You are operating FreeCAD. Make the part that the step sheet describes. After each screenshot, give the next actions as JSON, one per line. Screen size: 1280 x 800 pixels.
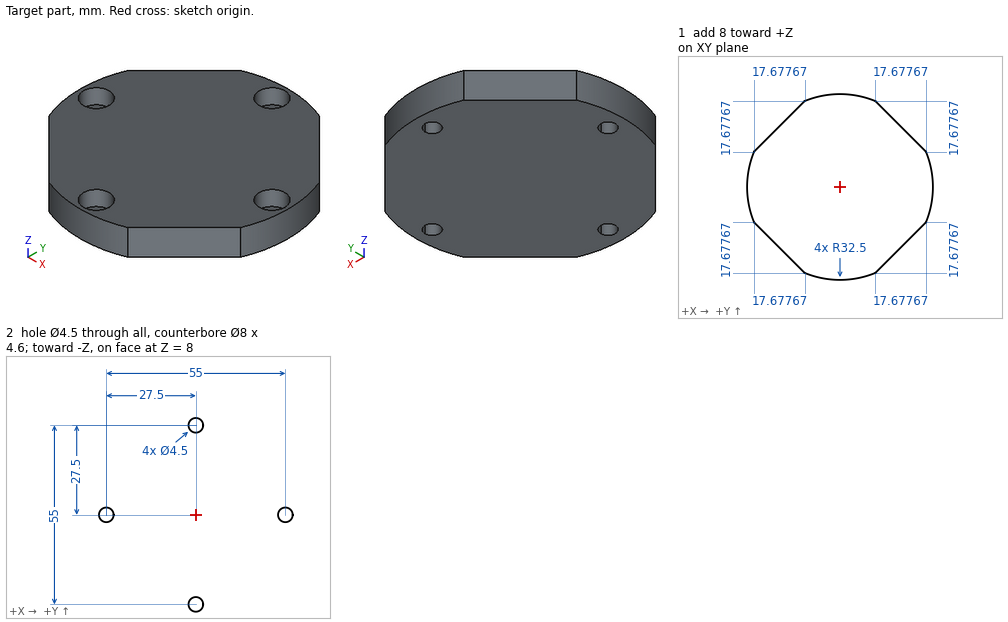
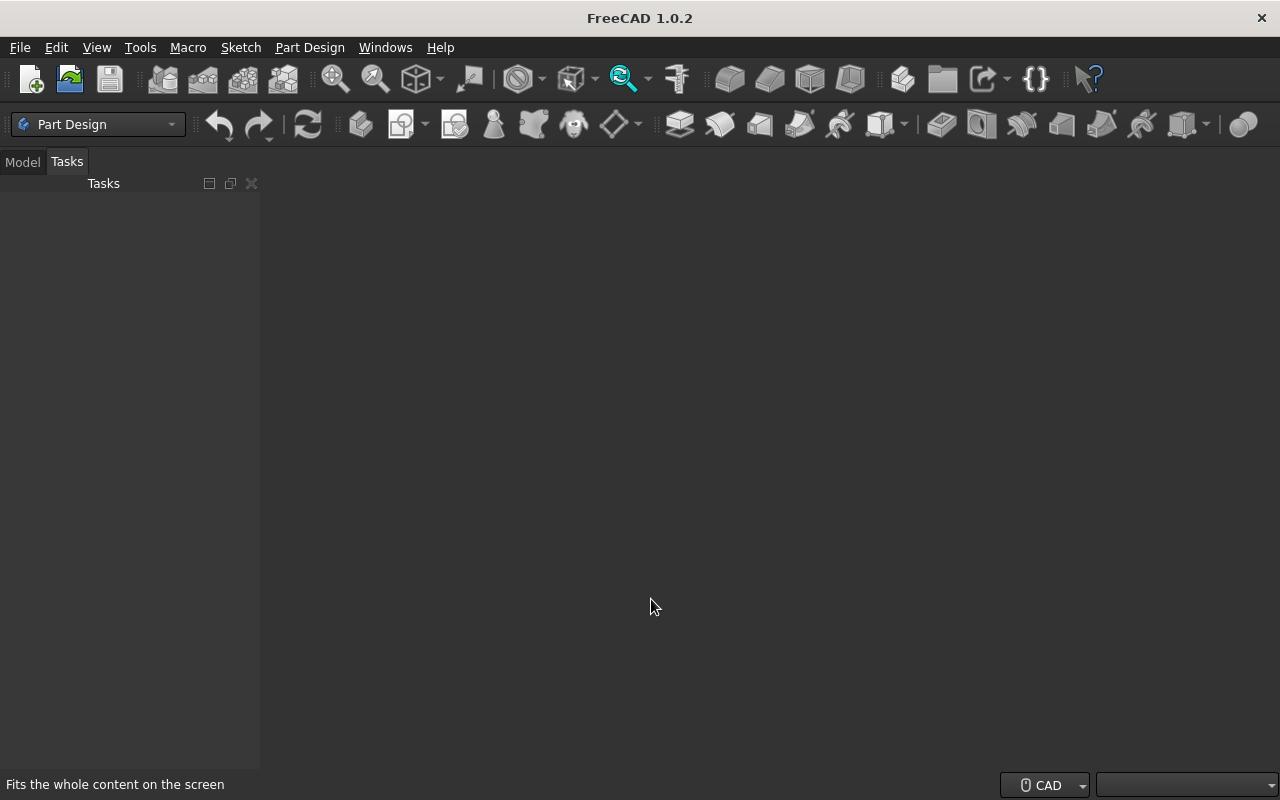
{"action": "left_click", "coordinate": [30, 80]}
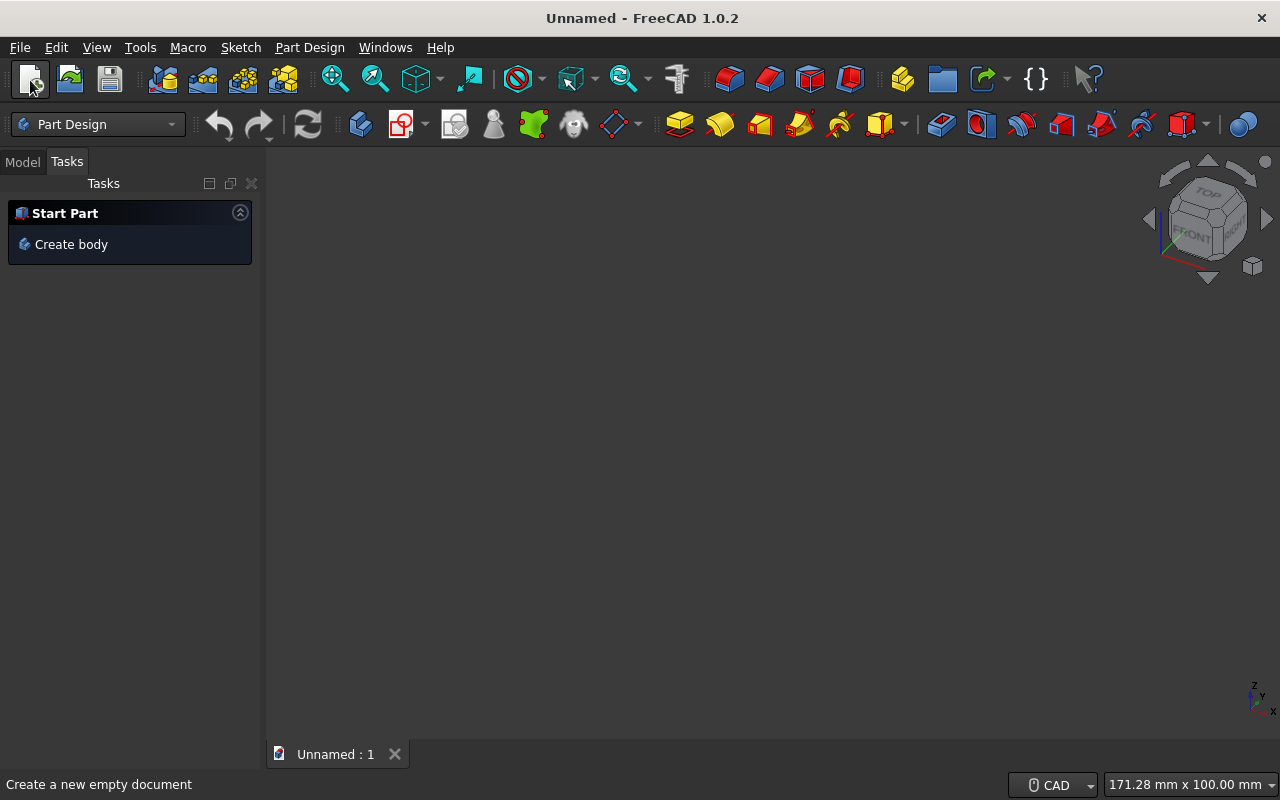
{"action": "left_click", "coordinate": [402, 124]}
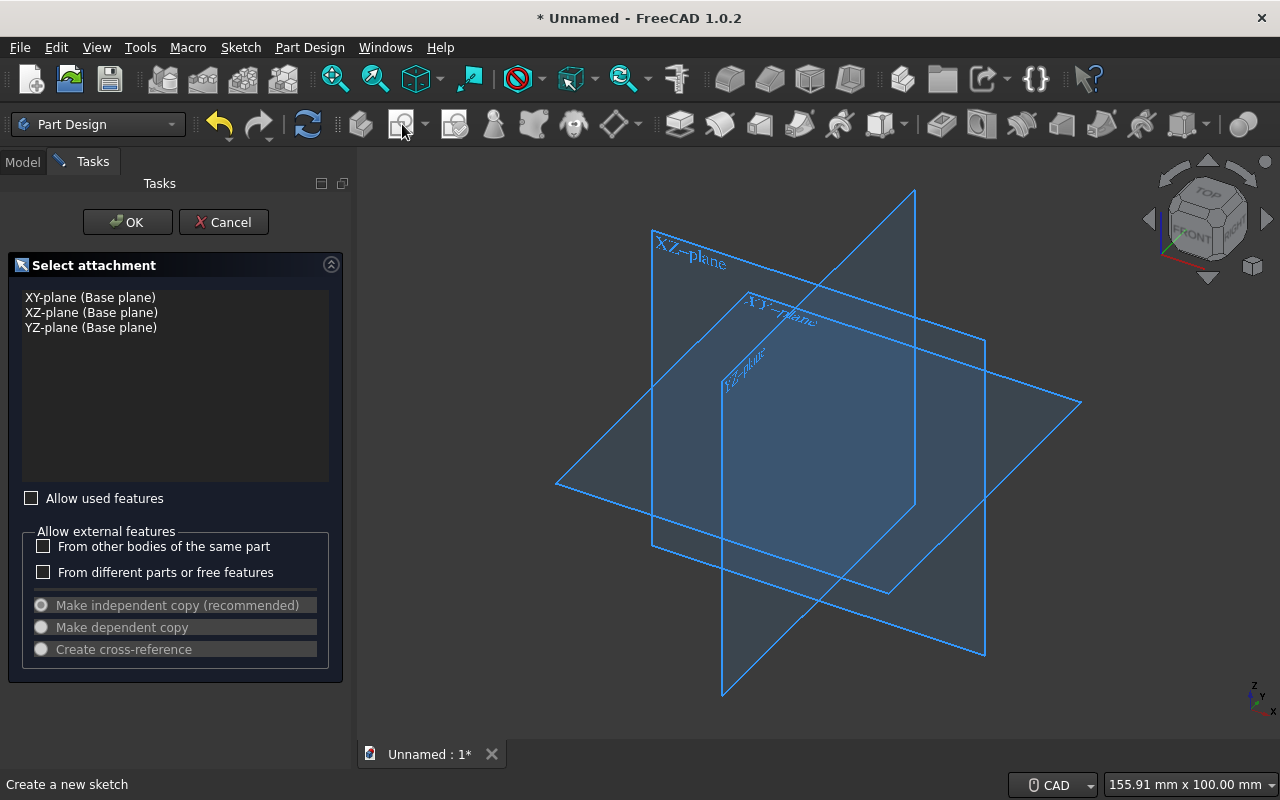
{"action": "left_click", "coordinate": [82, 298]}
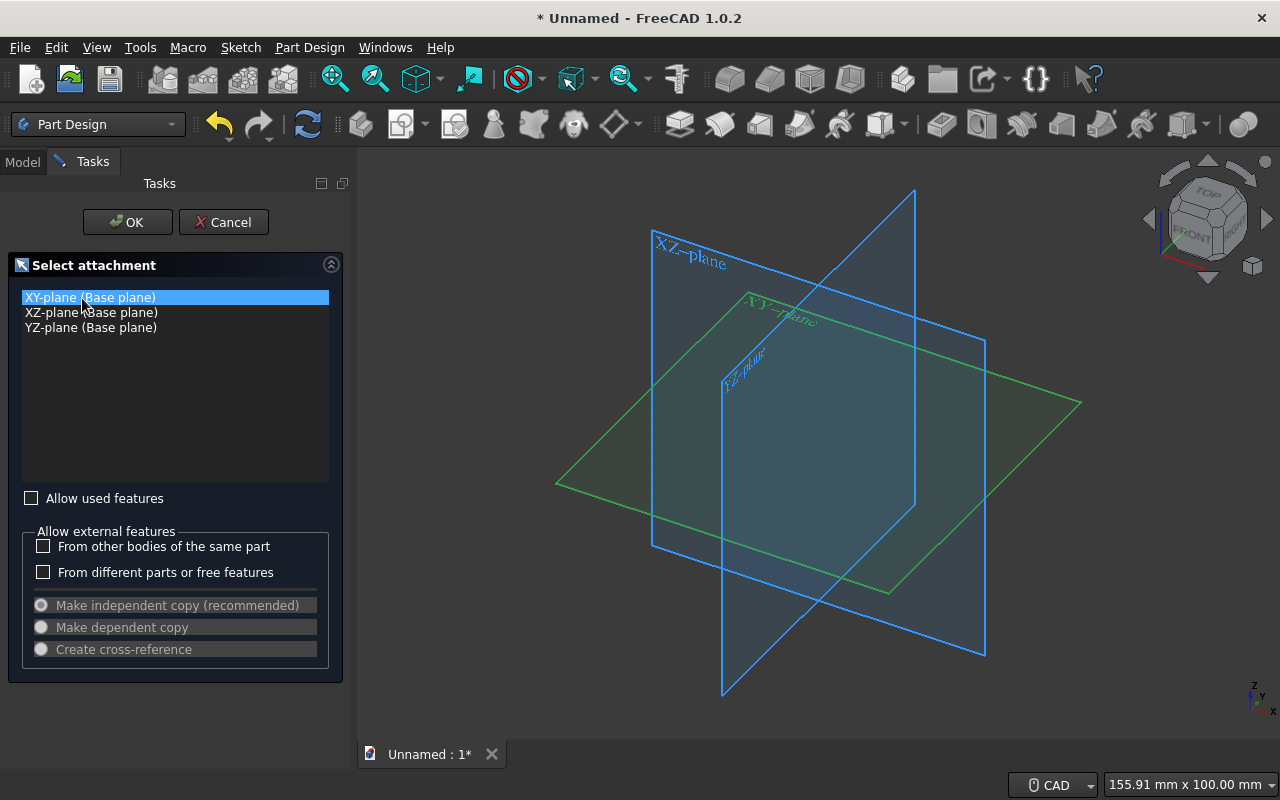
{"action": "left_click", "coordinate": [128, 222]}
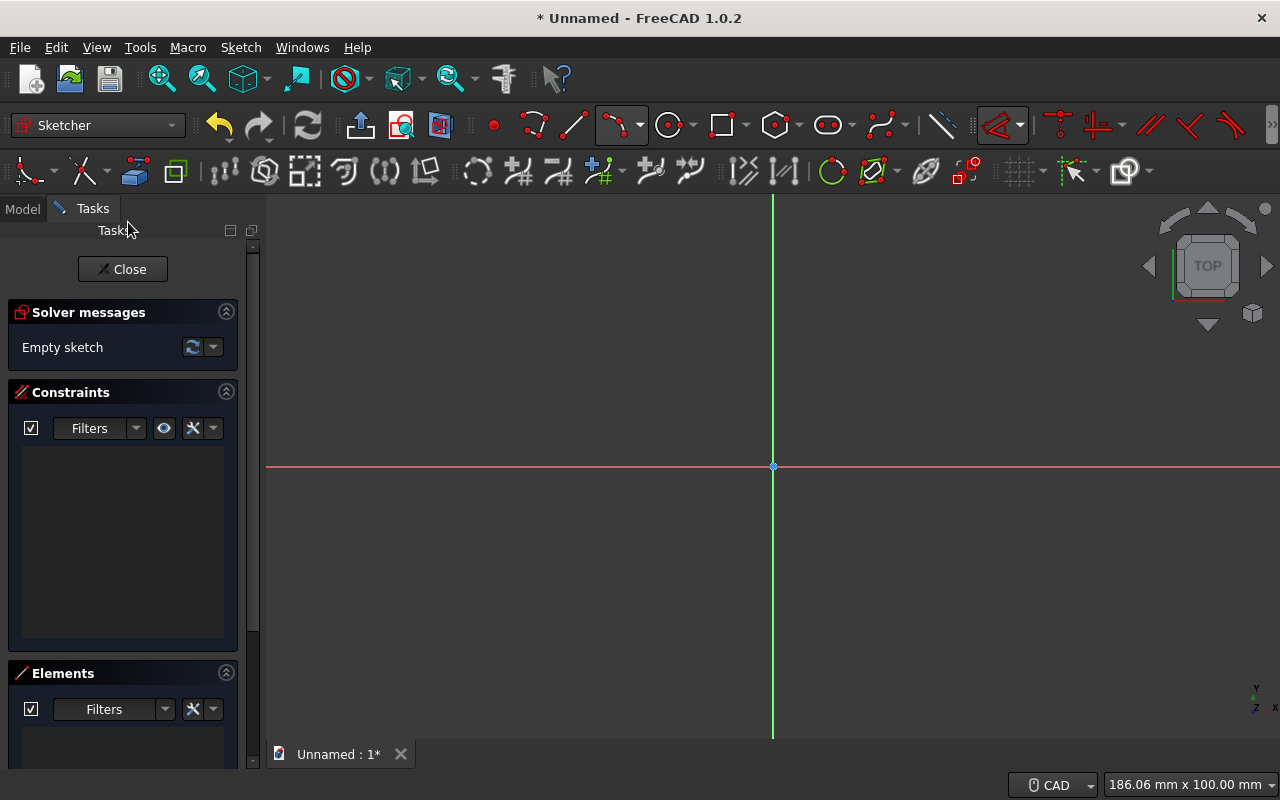
{"action": "left_click", "coordinate": [574, 126]}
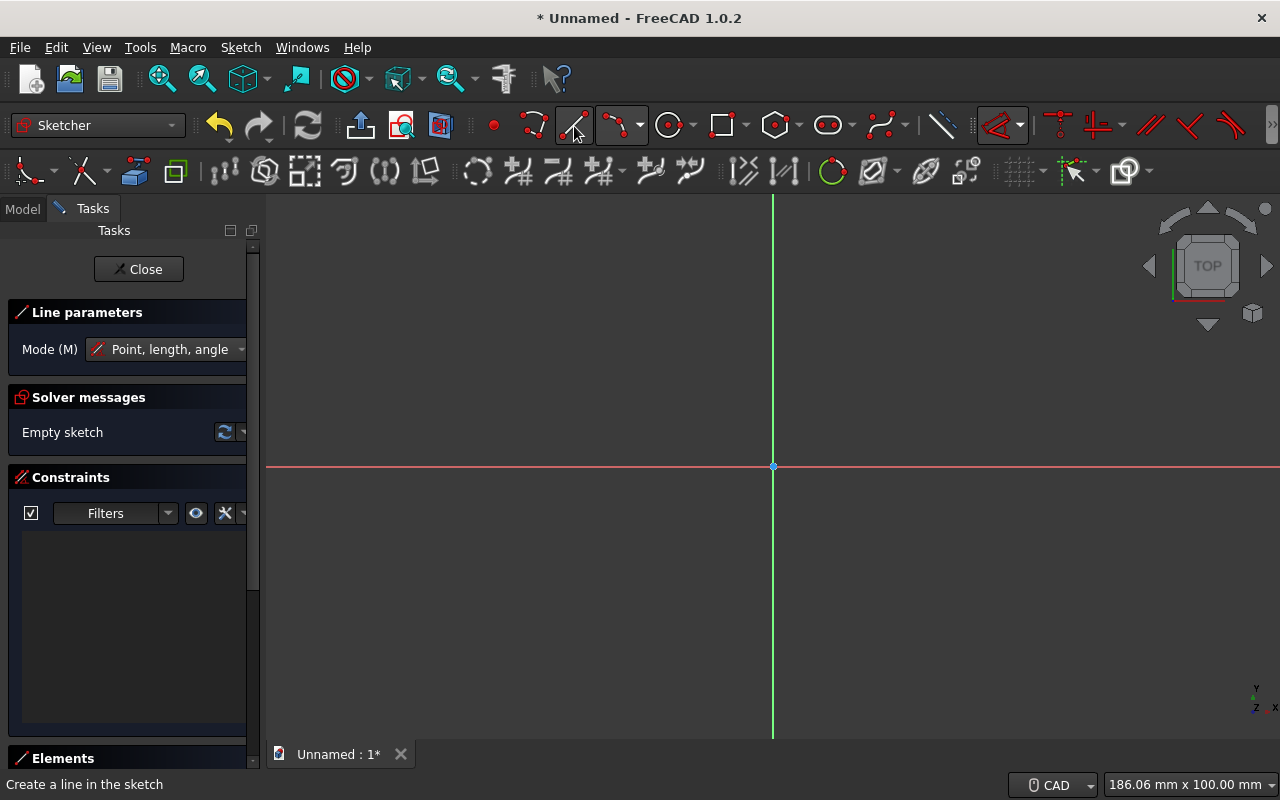
{"action": "left_click", "coordinate": [609, 534]}
{"action": "left_click", "coordinate": [706, 630]}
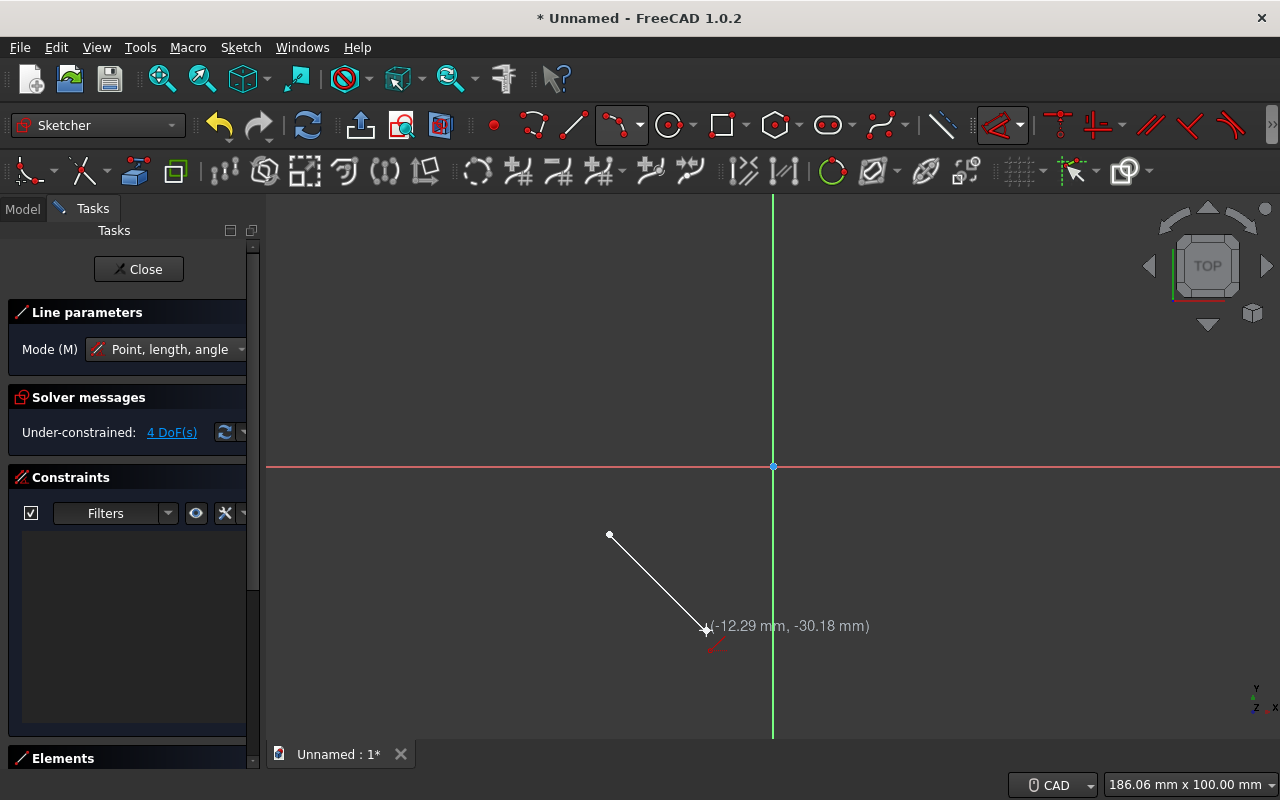
{"action": "left_click", "coordinate": [840, 630]}
{"action": "left_click", "coordinate": [937, 534]}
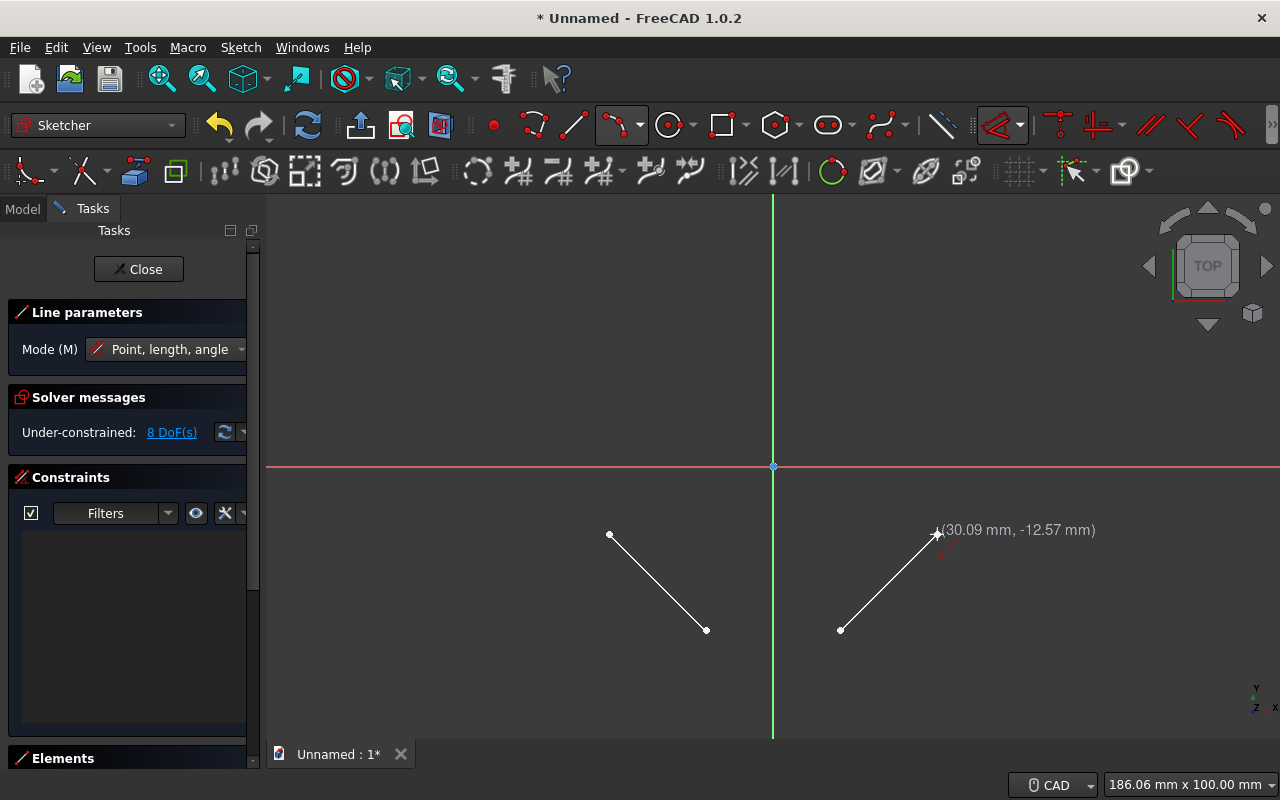
{"action": "left_click", "coordinate": [937, 399]}
{"action": "left_click", "coordinate": [840, 303]}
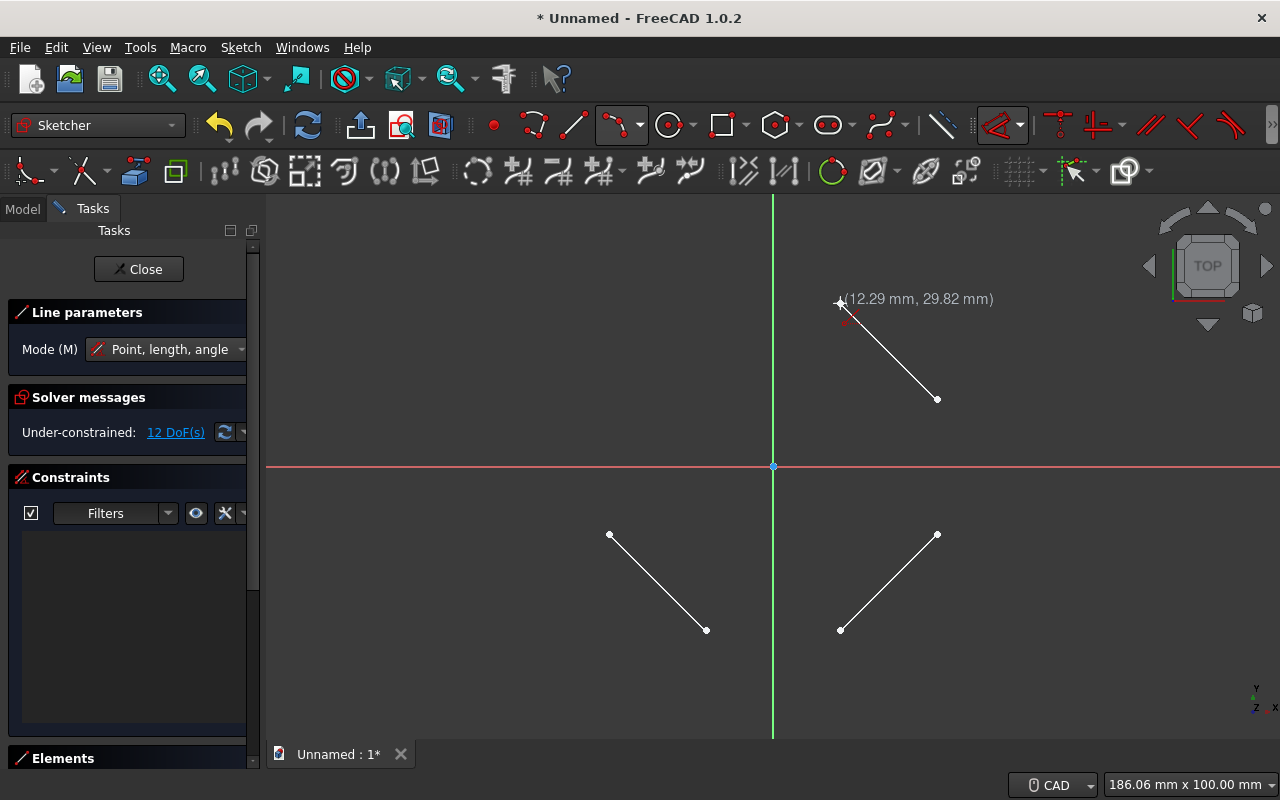
{"action": "left_click", "coordinate": [706, 303]}
{"action": "left_click", "coordinate": [609, 399]}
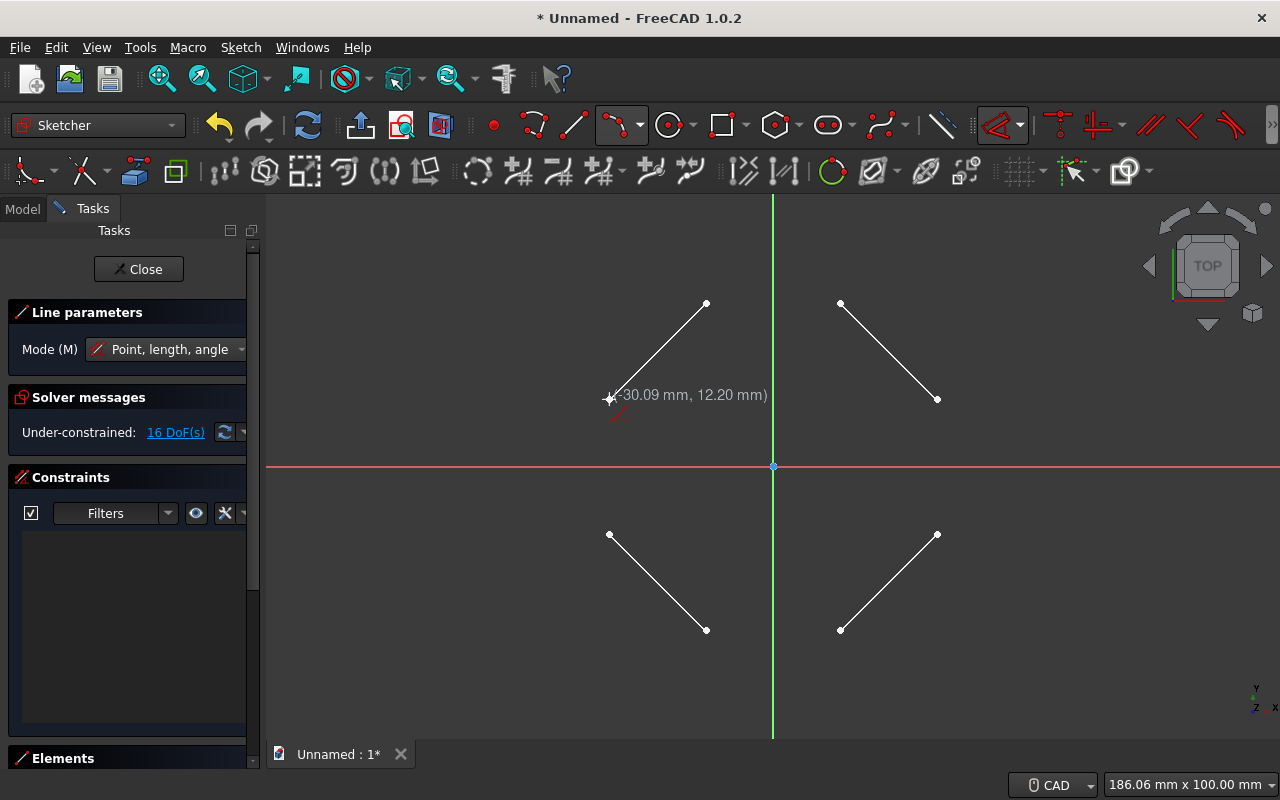
{"action": "left_click", "coordinate": [616, 126]}